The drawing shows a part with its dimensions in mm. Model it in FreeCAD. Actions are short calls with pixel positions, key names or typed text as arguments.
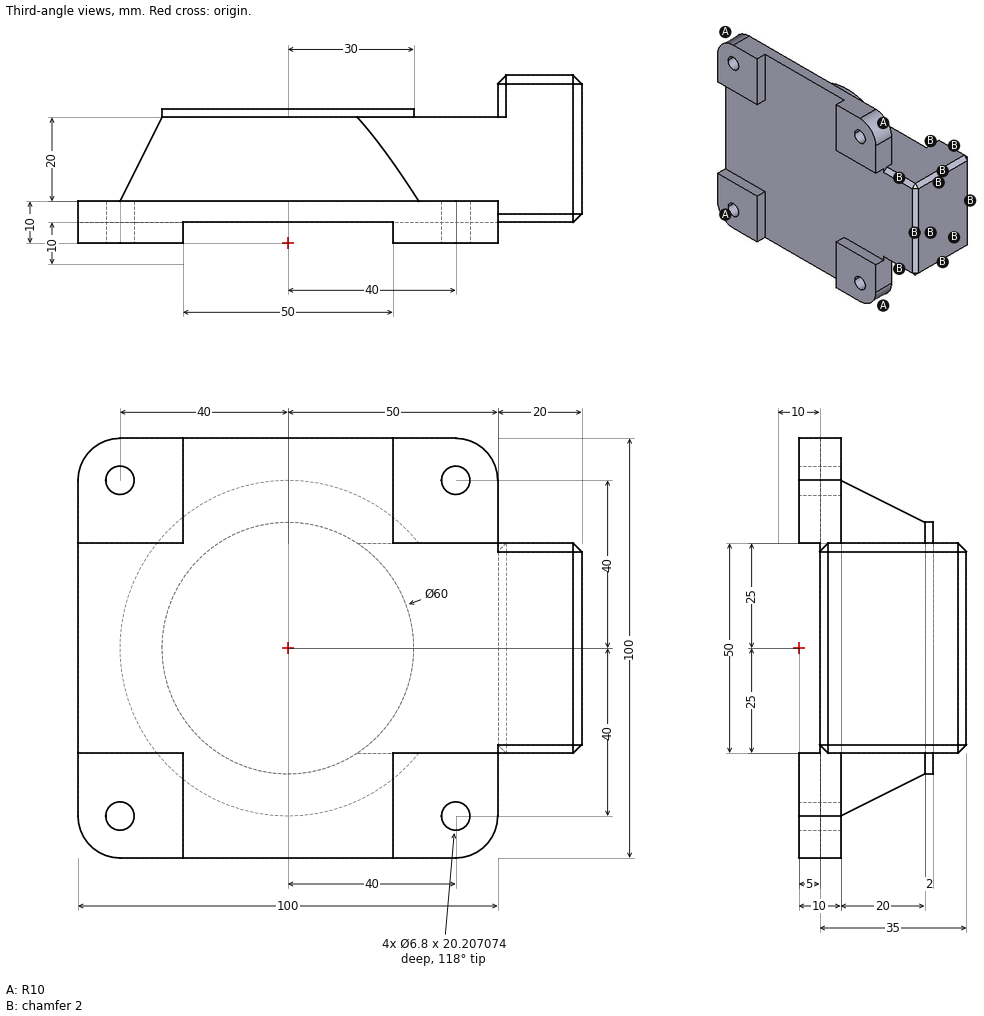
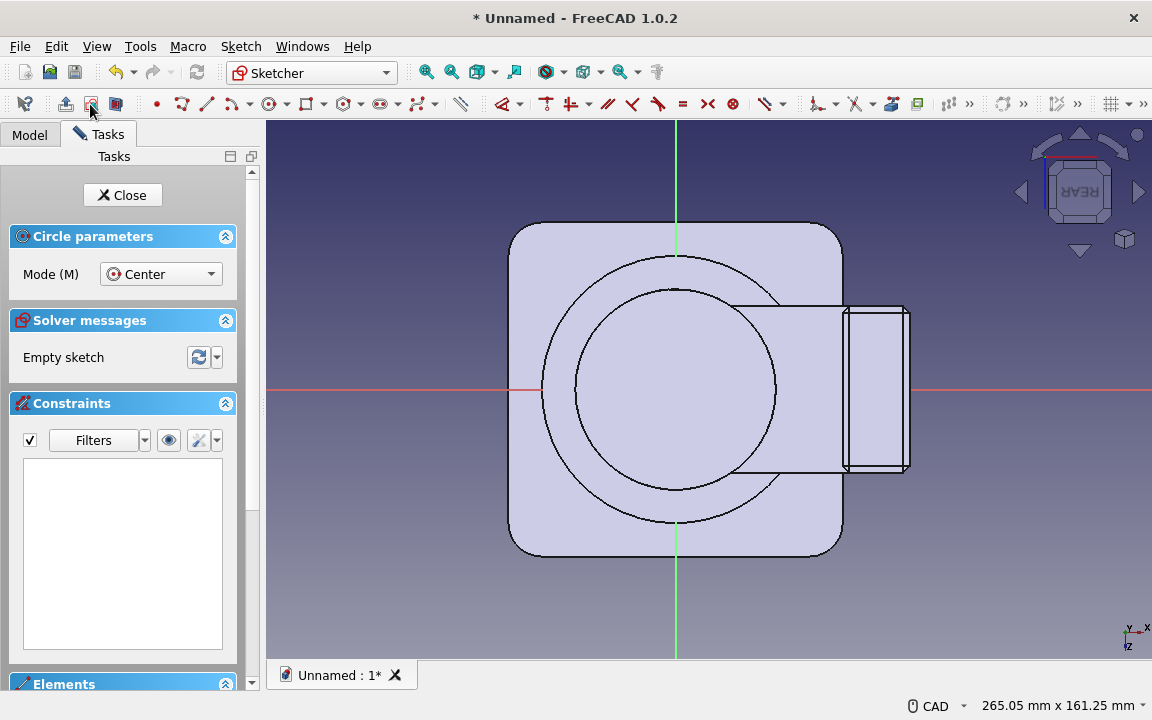
scroll(809, 256, up, 4)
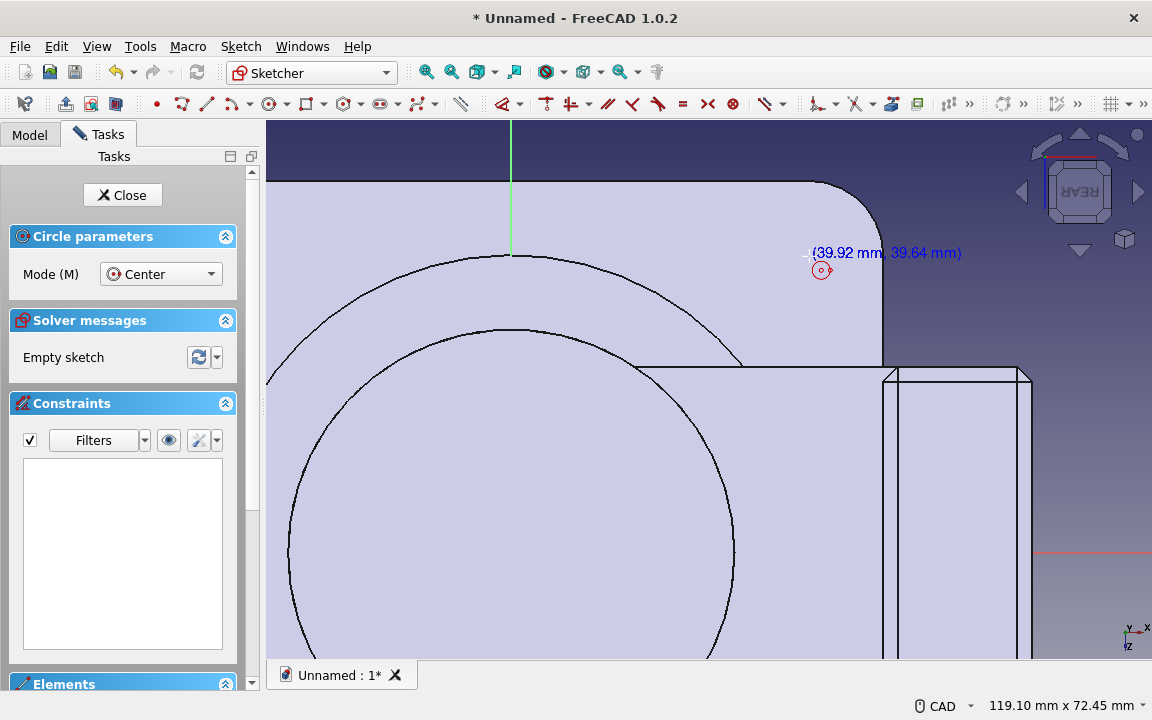
click(809, 255)
click(827, 237)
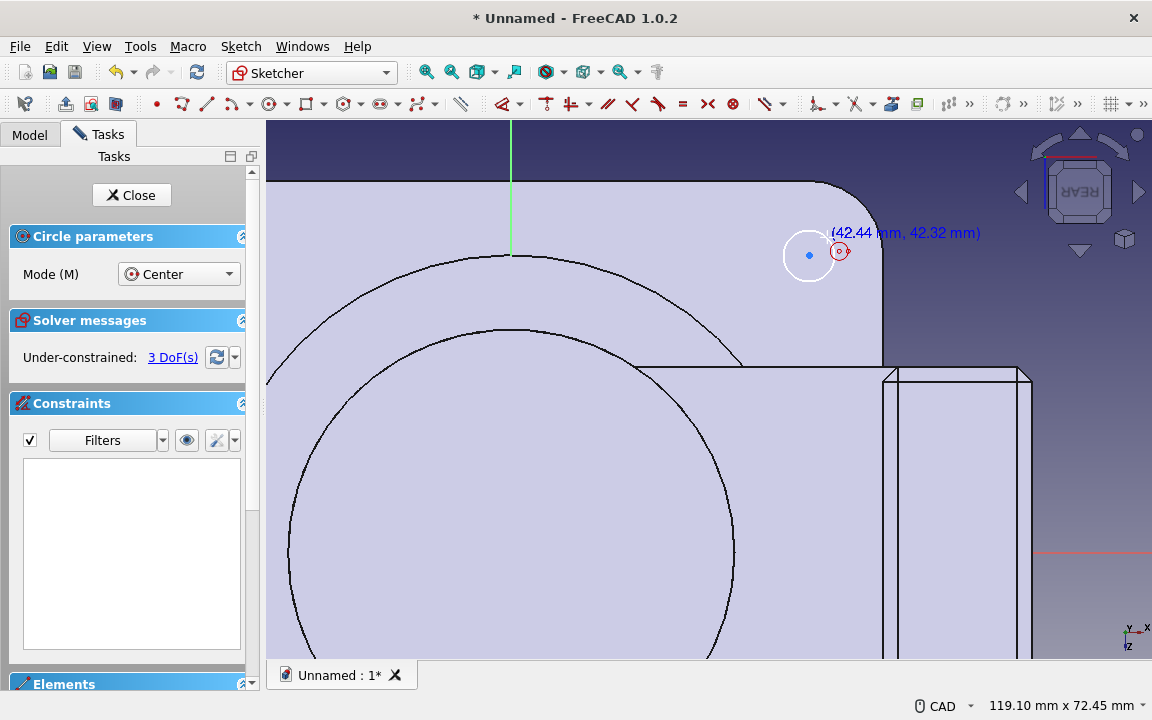
scroll(798, 191, down, 3)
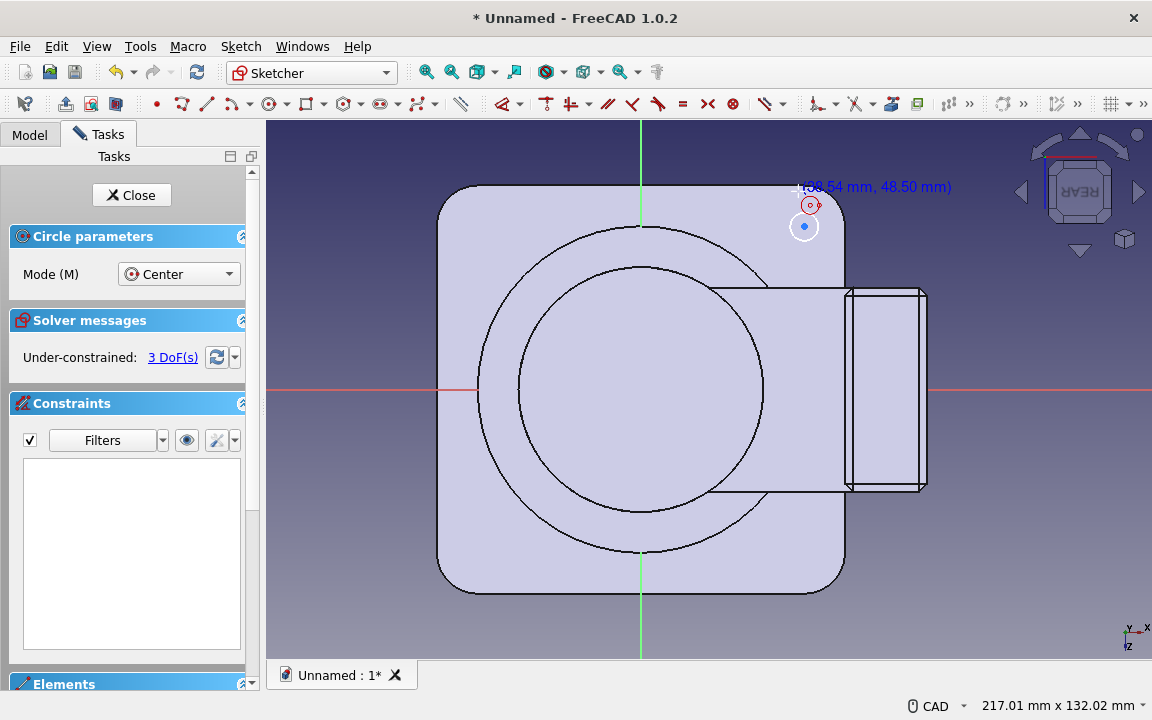
scroll(804, 553, up, 3)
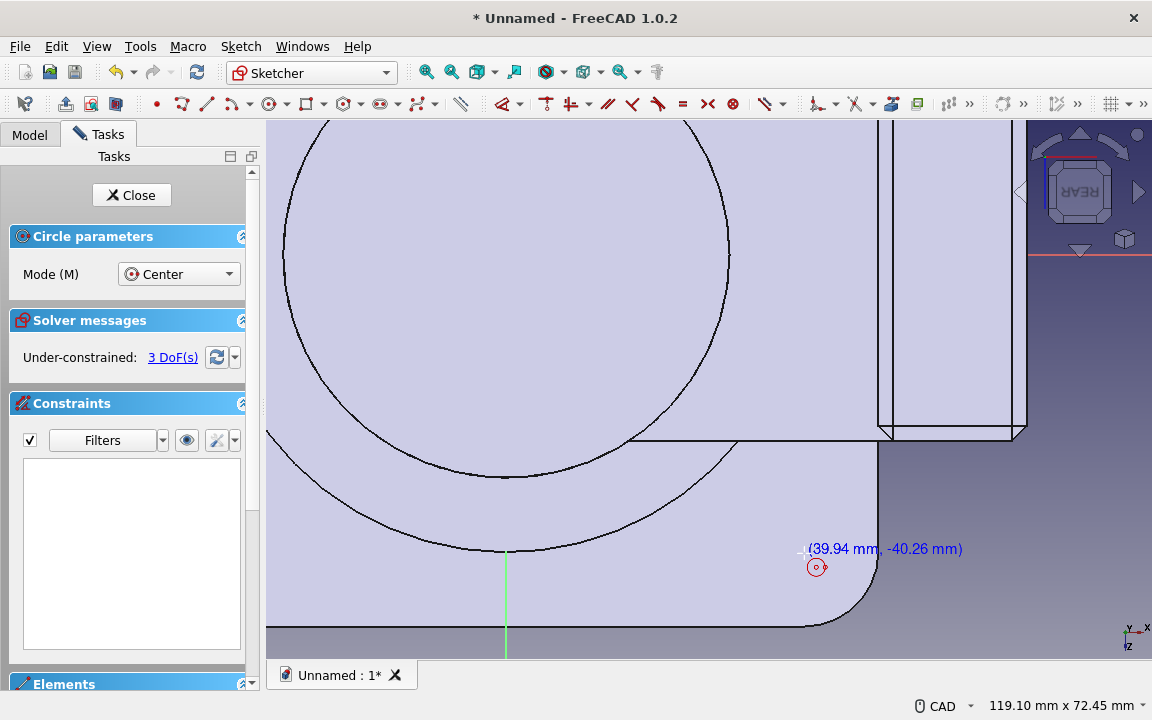
click(804, 552)
click(822, 534)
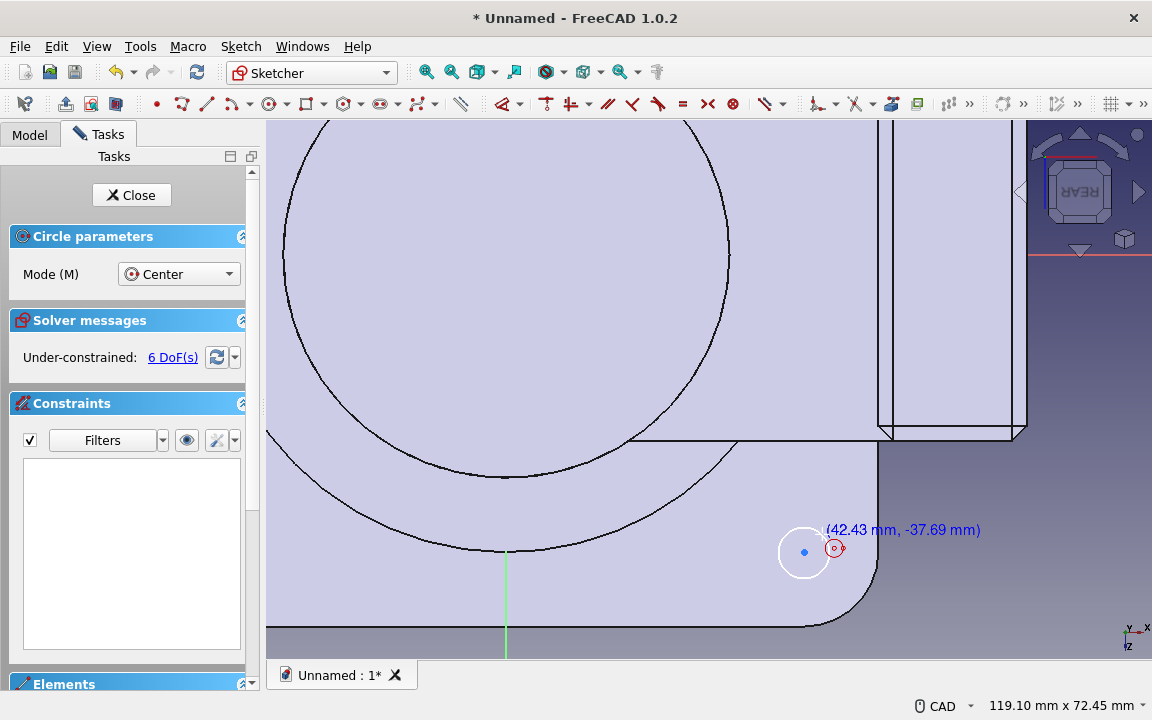
scroll(804, 554, down, 3)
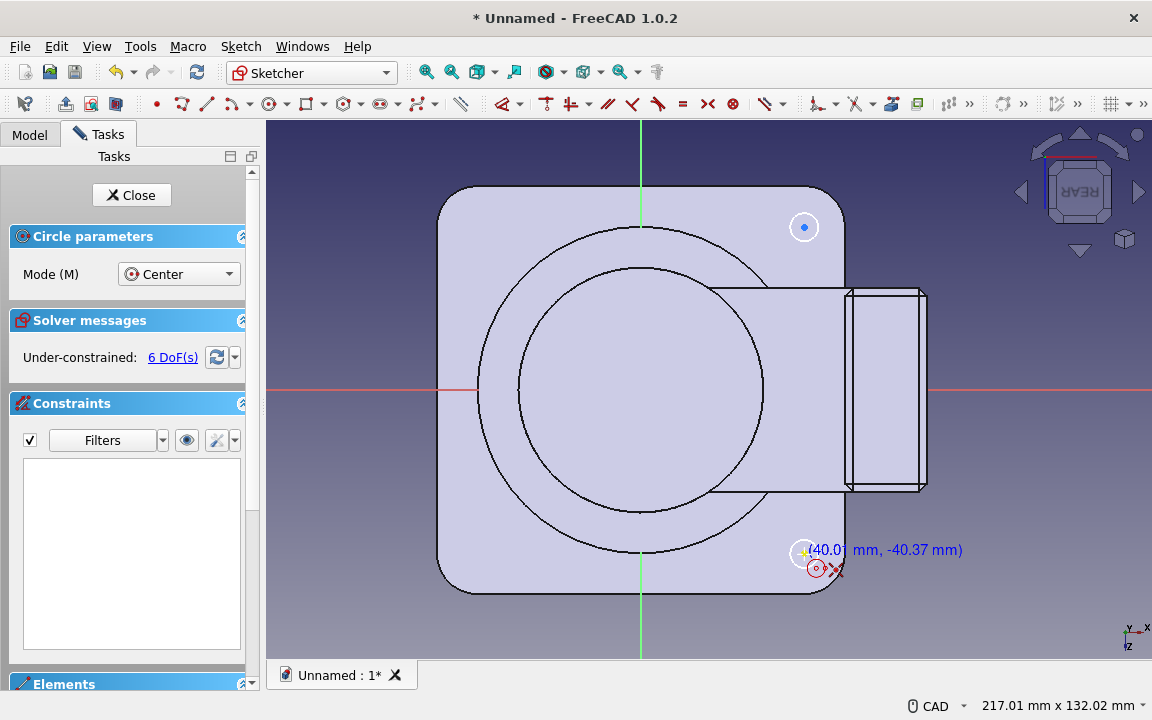
scroll(478, 553, up, 3)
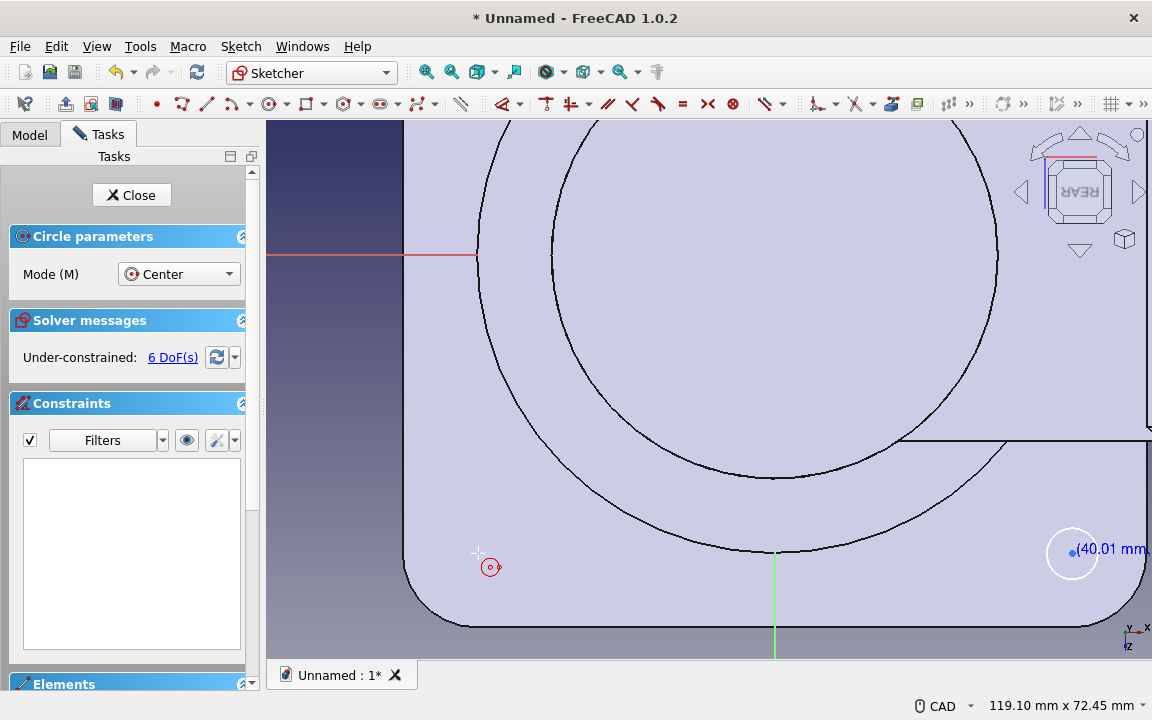
click(477, 553)
click(495, 535)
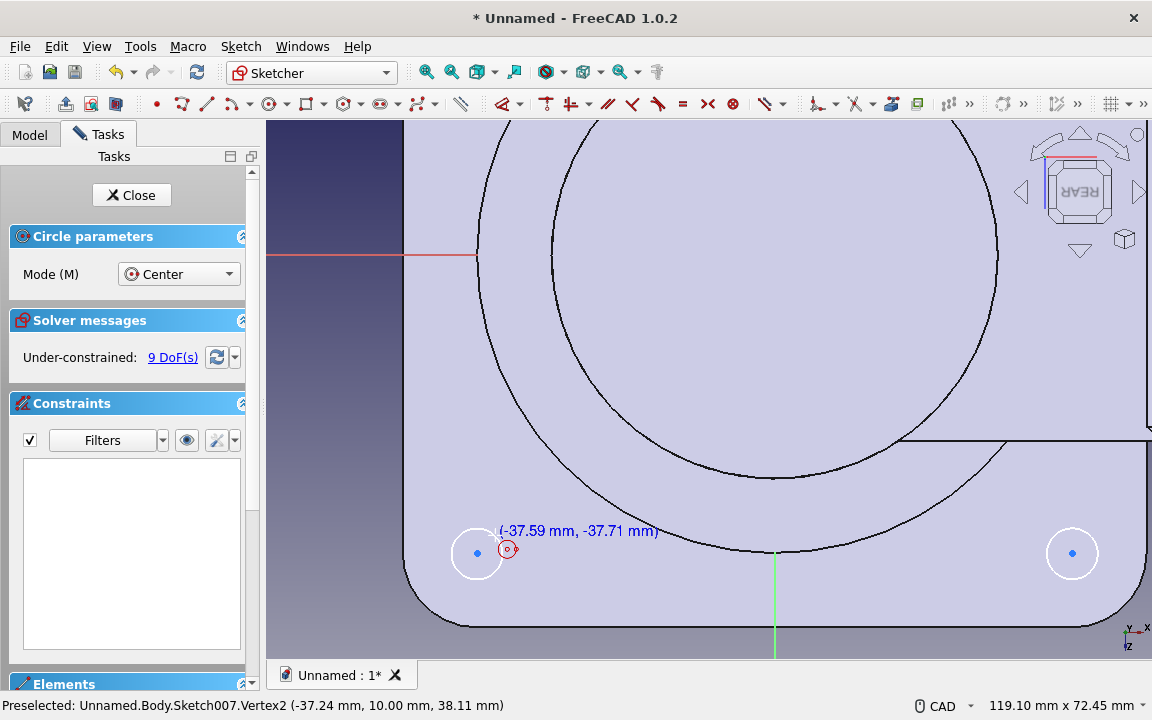
scroll(477, 553, down, 3)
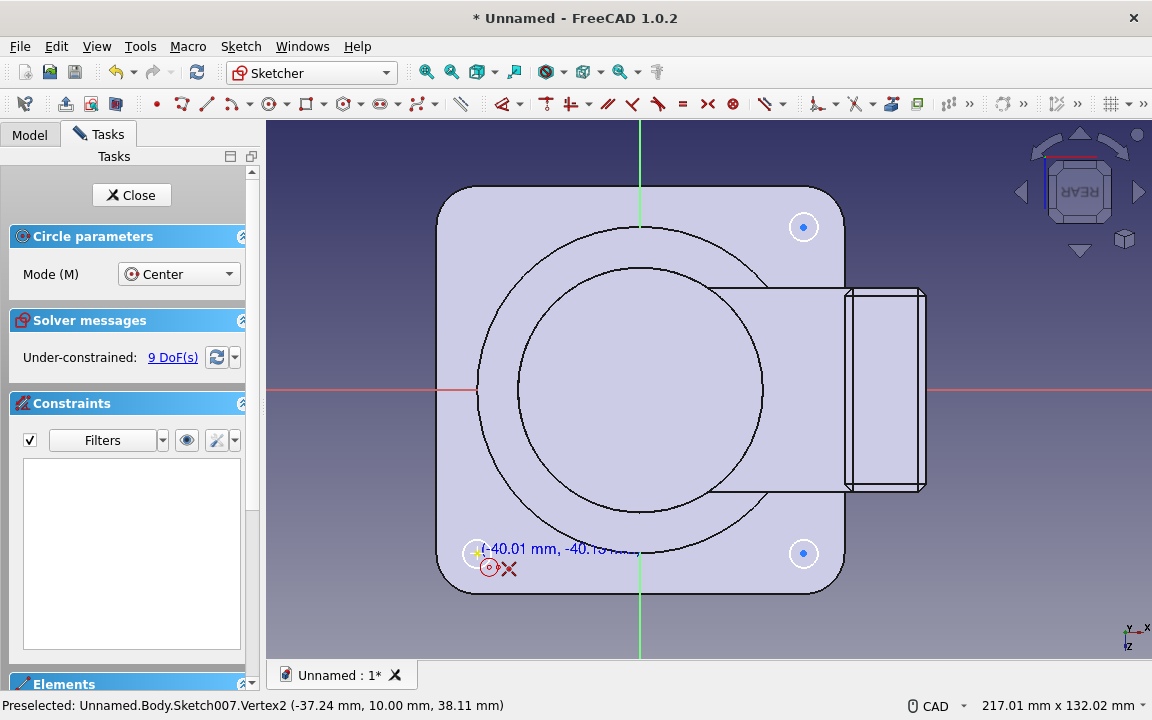
scroll(477, 227, up, 3)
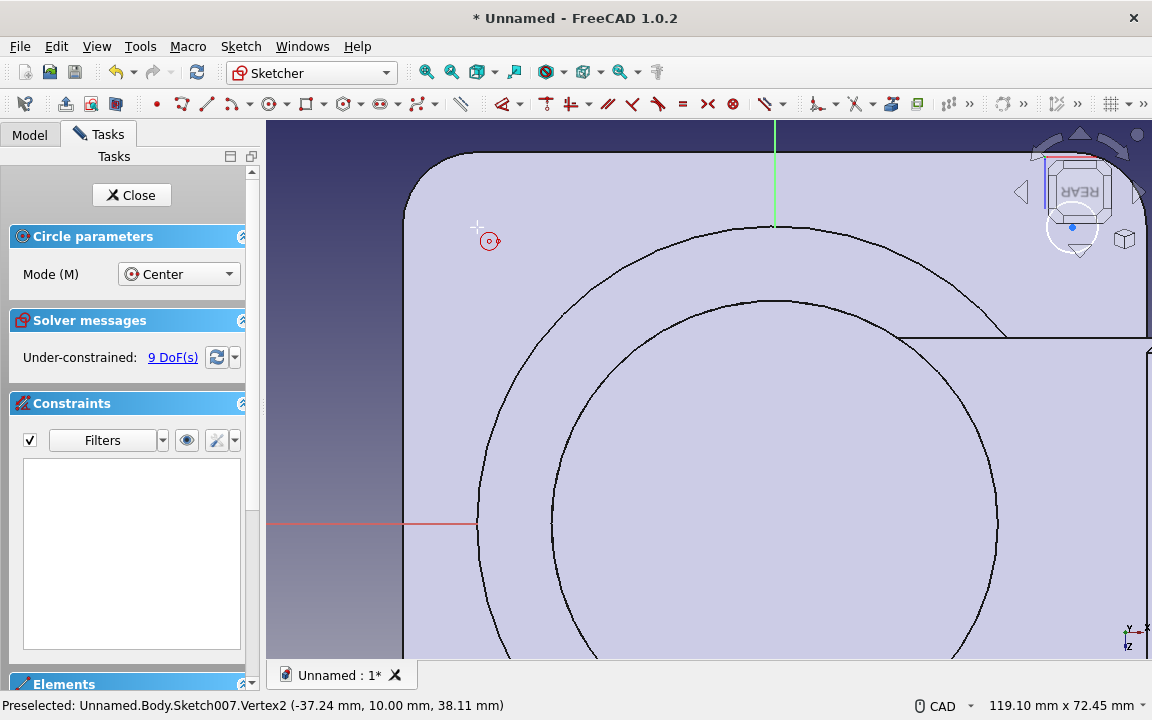
click(477, 226)
click(495, 209)
key(Escape)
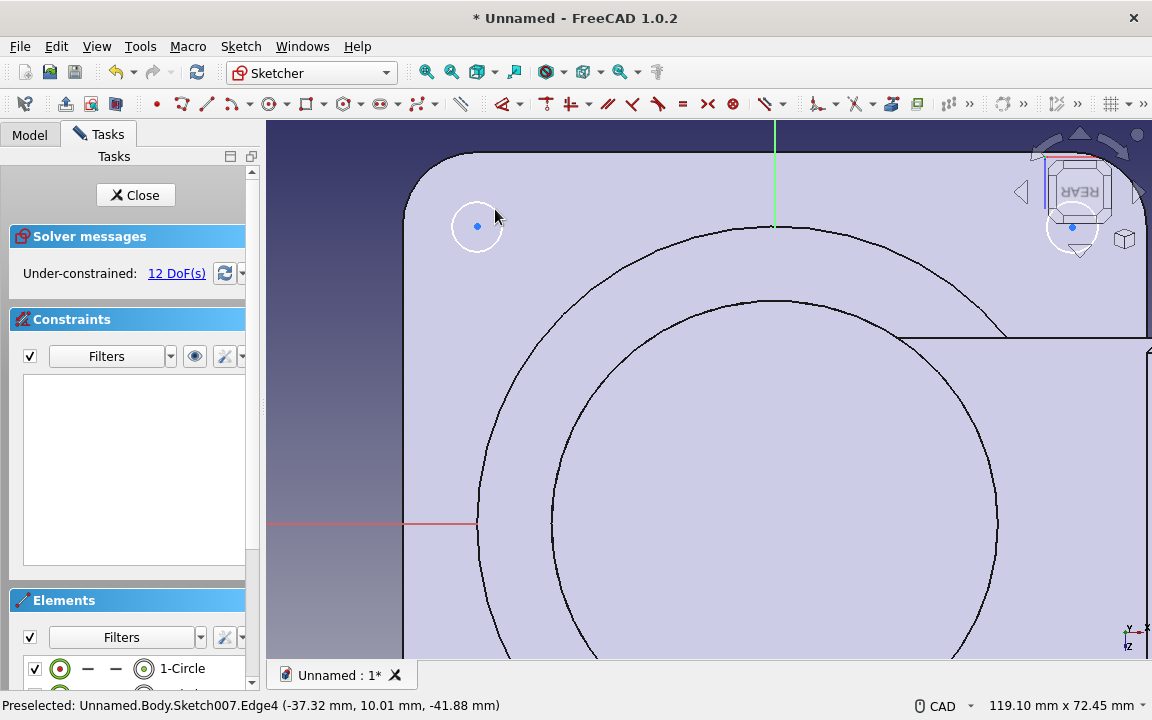
scroll(477, 226, down, 3)